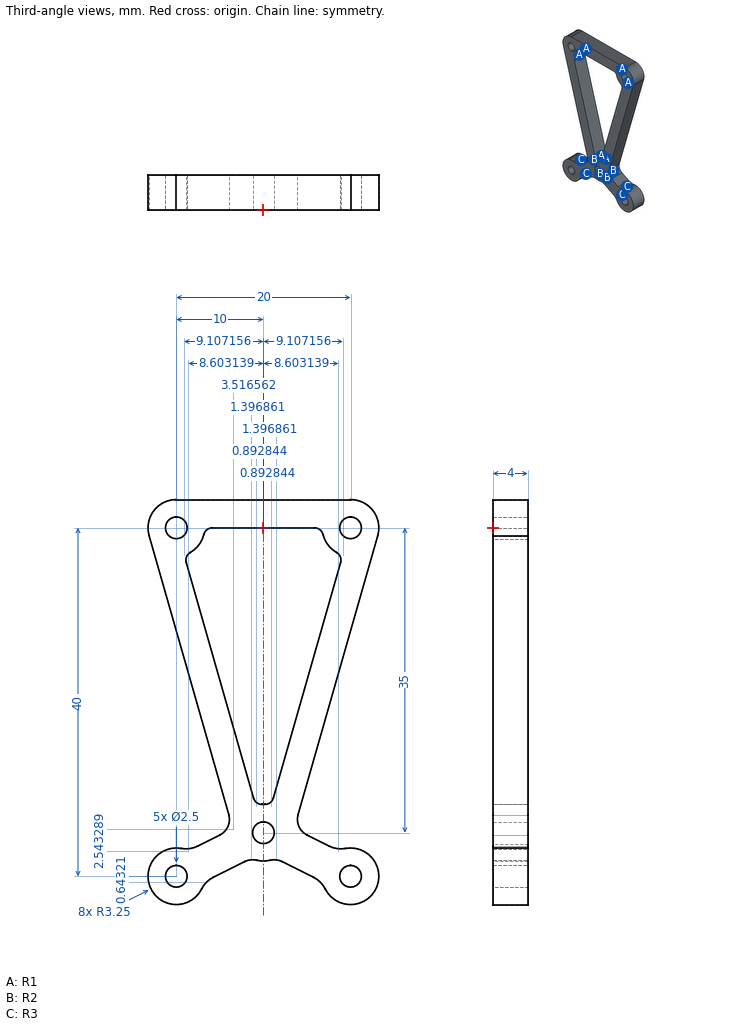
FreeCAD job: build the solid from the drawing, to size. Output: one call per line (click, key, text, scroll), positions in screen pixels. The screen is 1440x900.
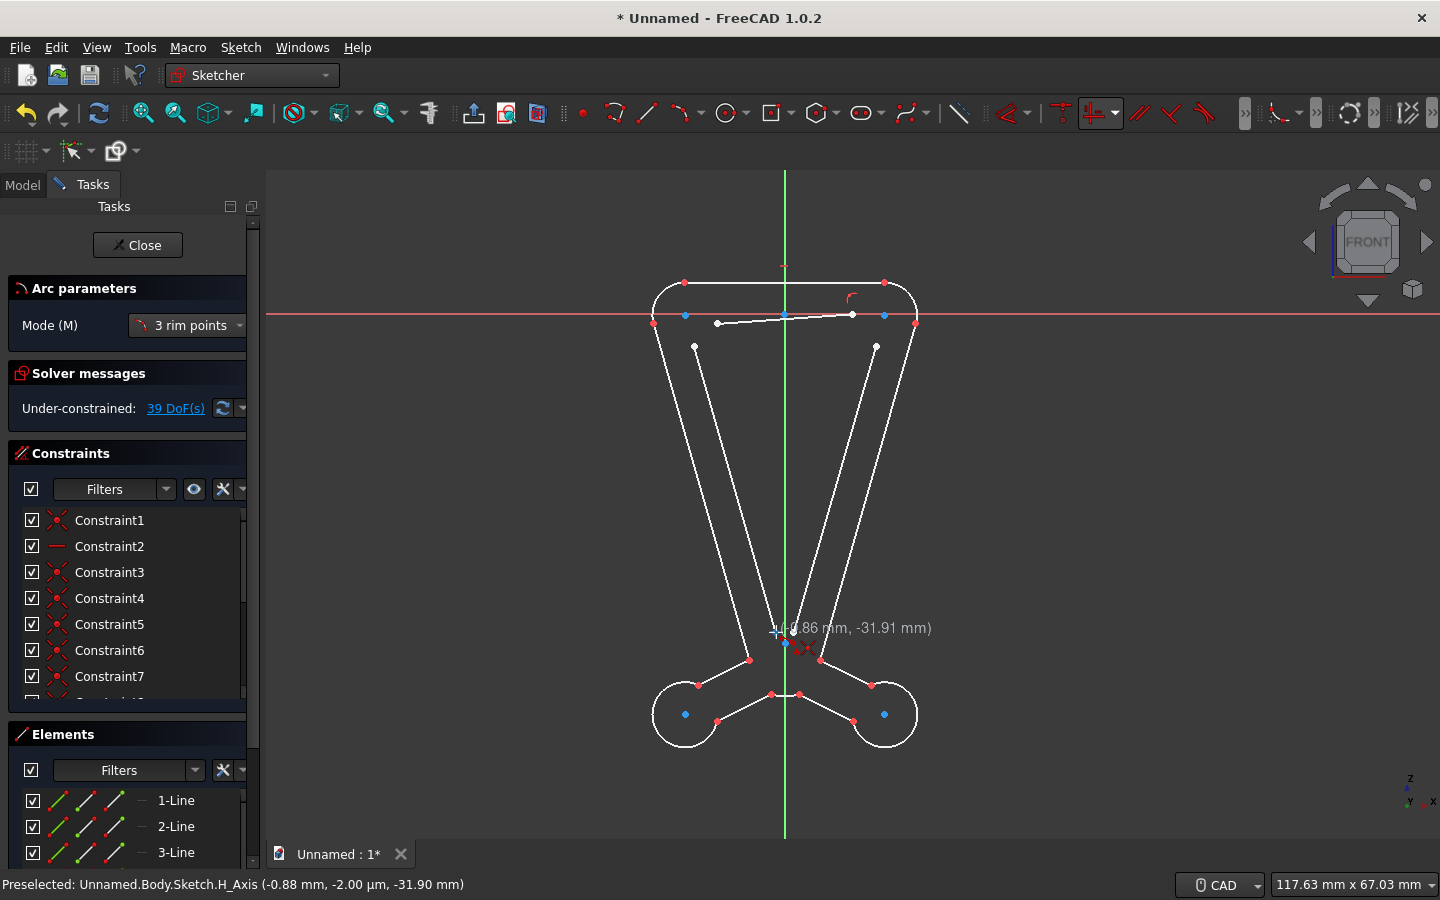
click(876, 347)
click(852, 314)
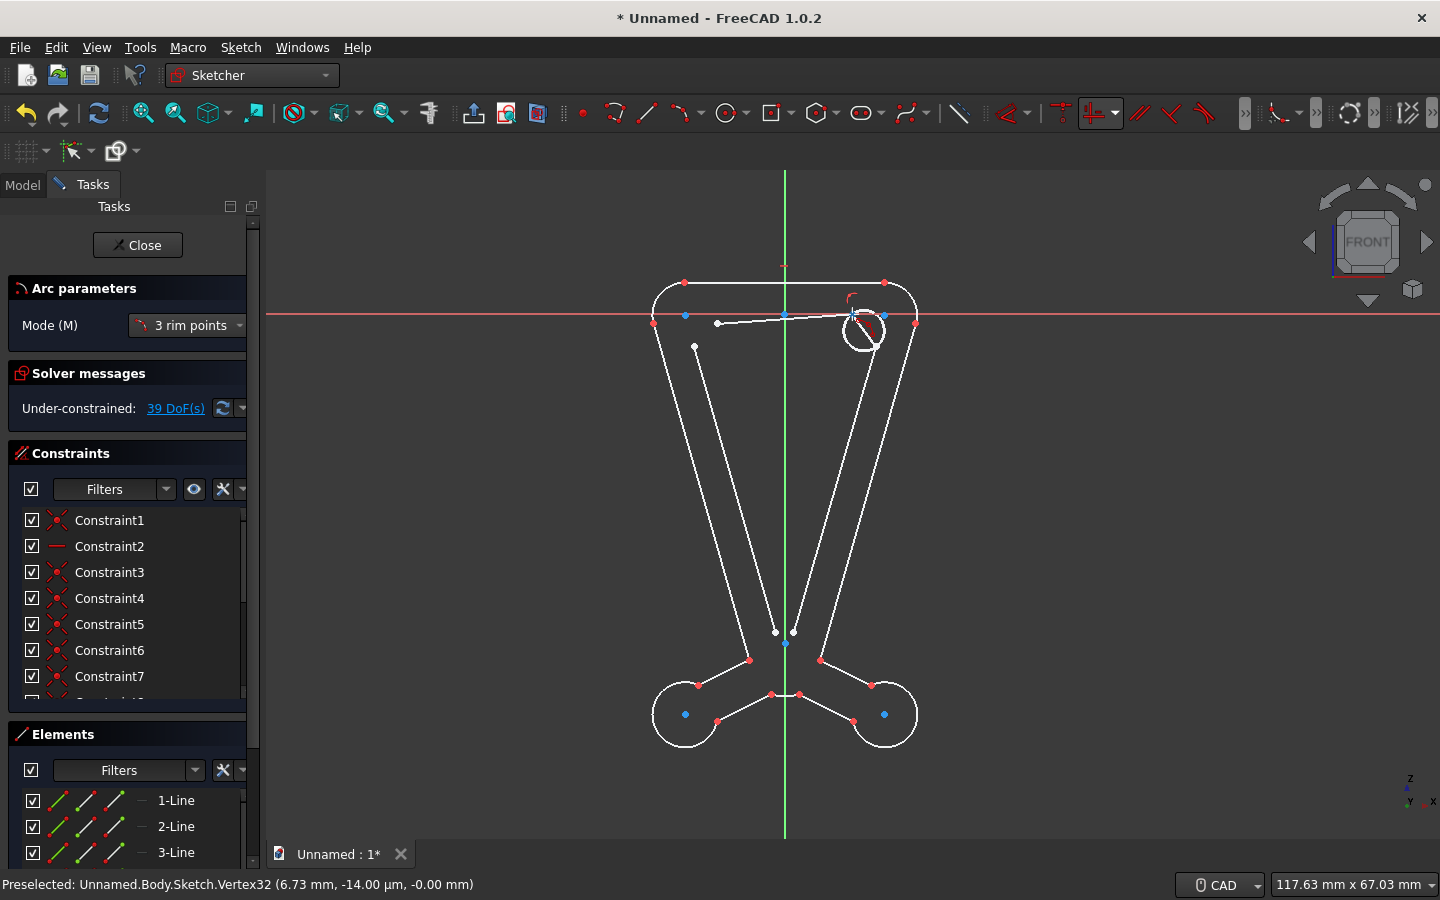
scroll(859, 334, up, 5)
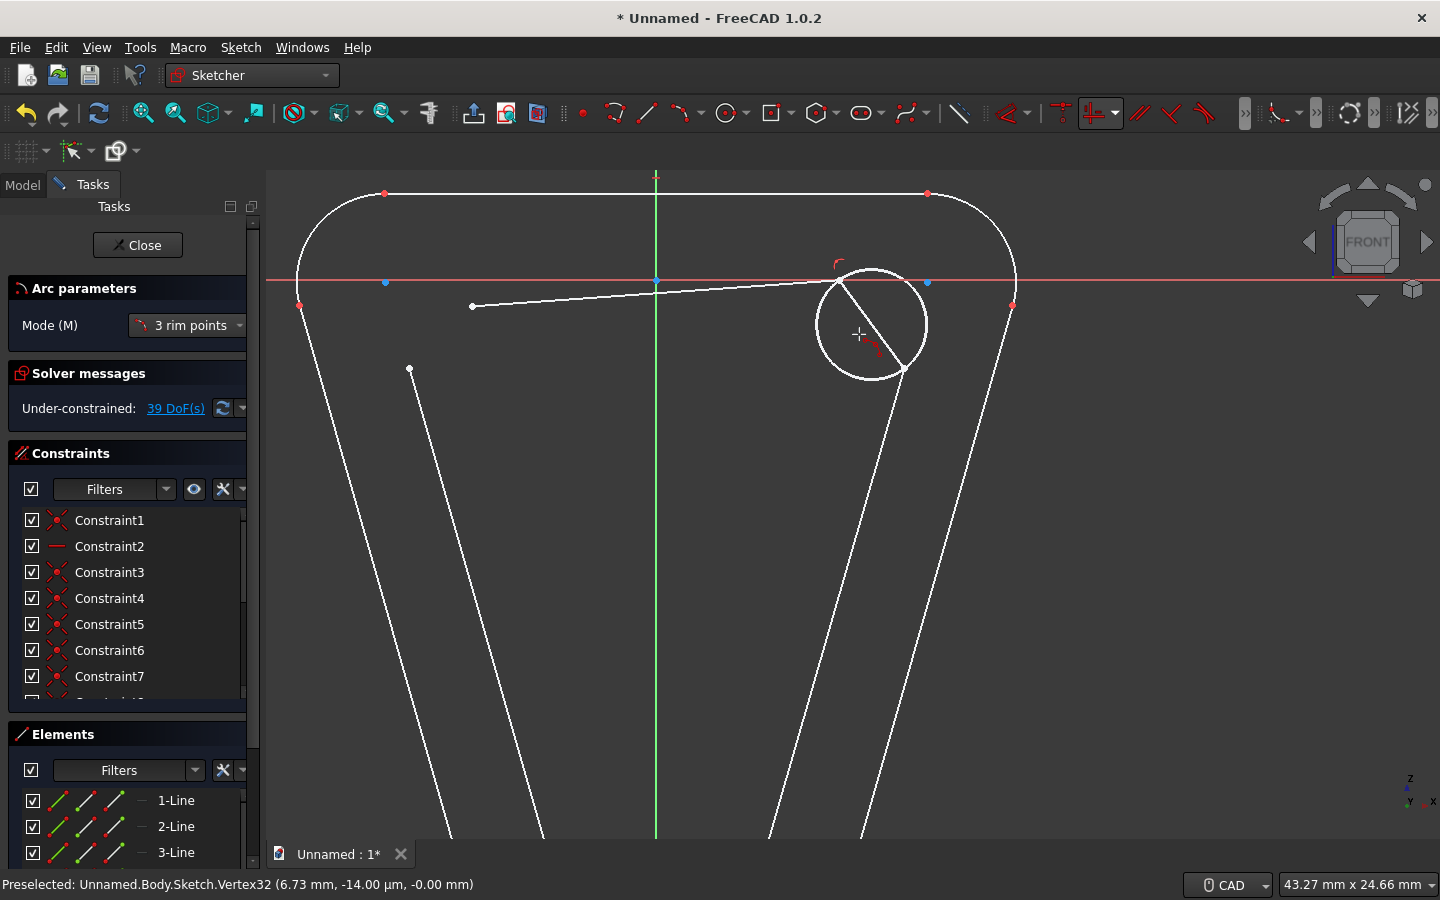
click(857, 333)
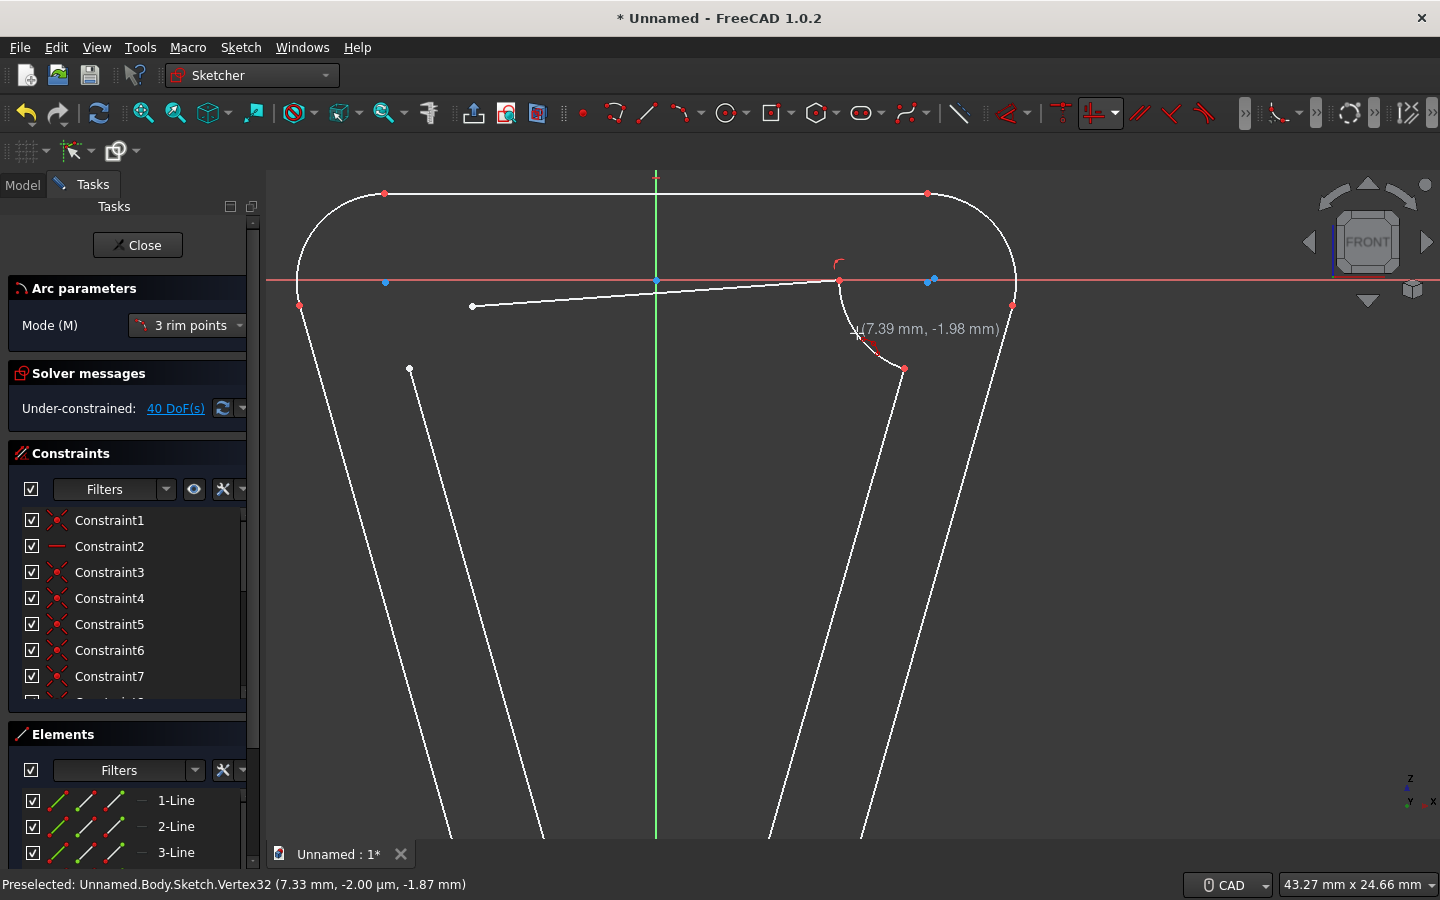
click(472, 306)
click(410, 369)
click(455, 333)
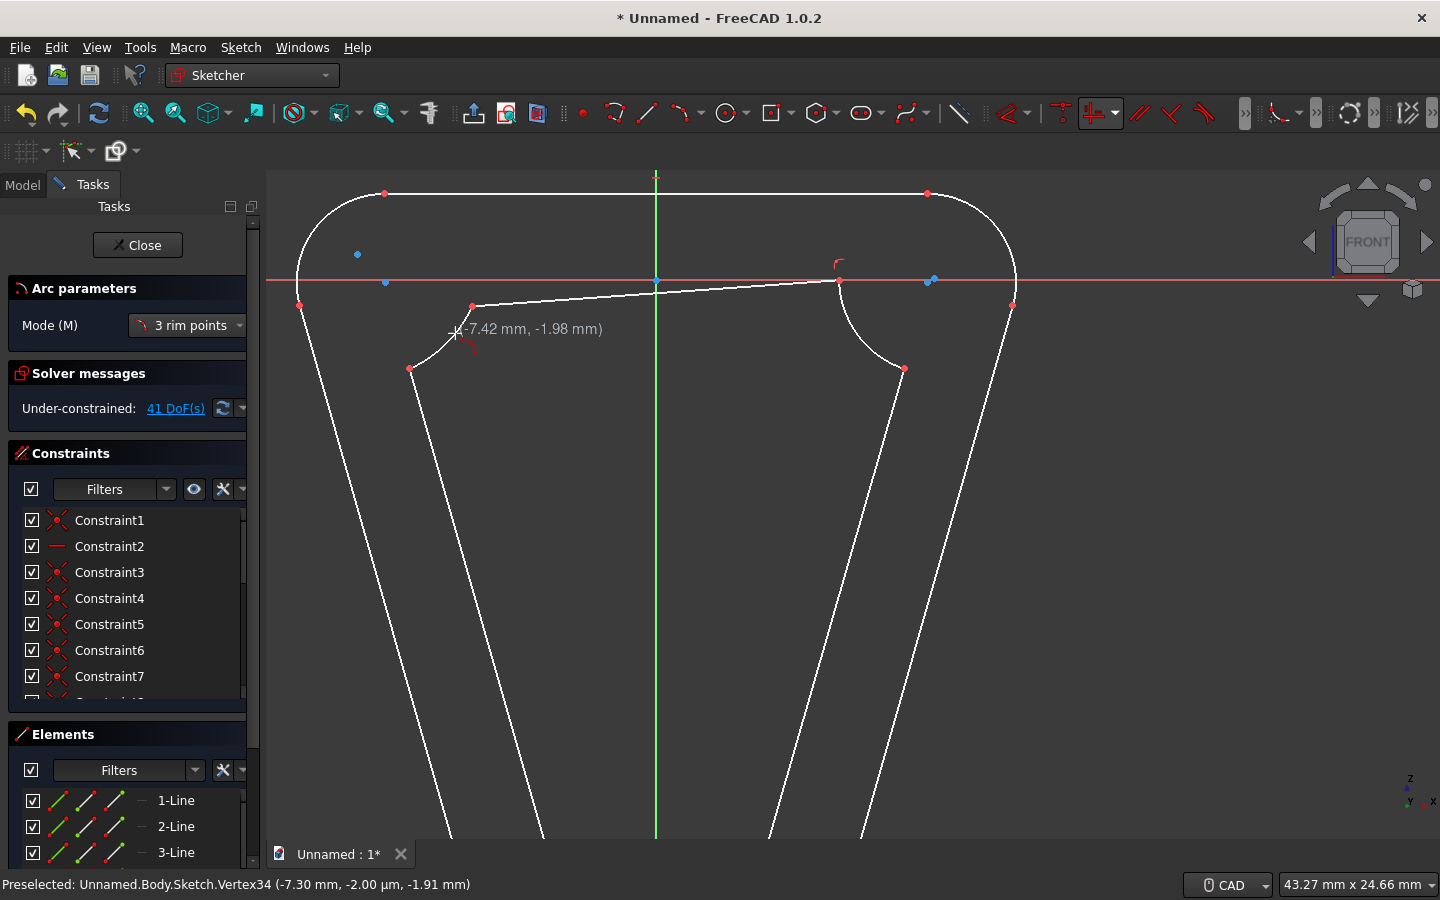
scroll(859, 333, down, 5)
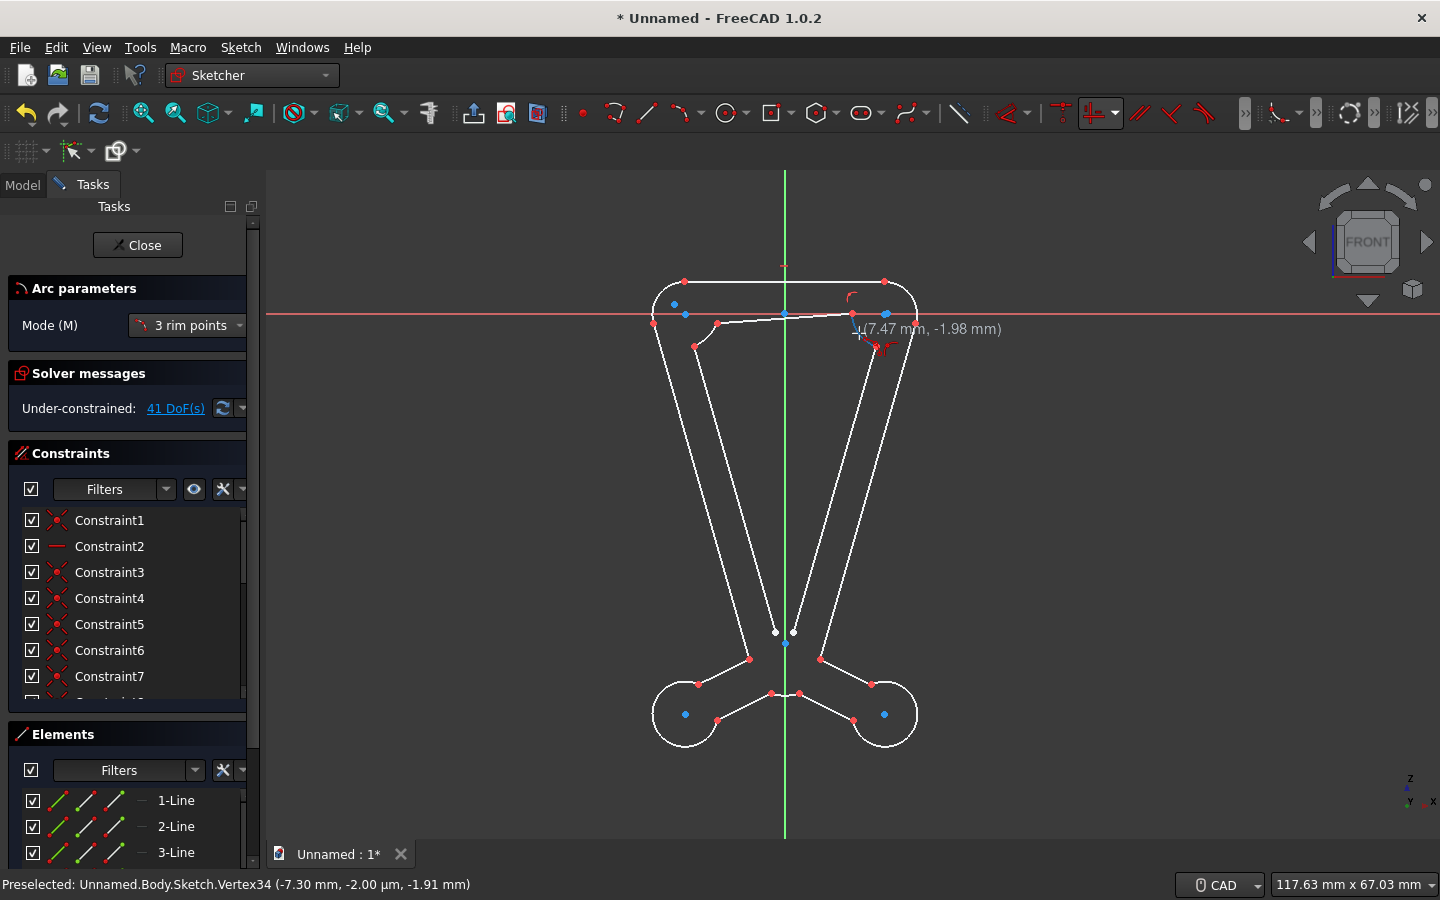
scroll(776, 632, up, 3)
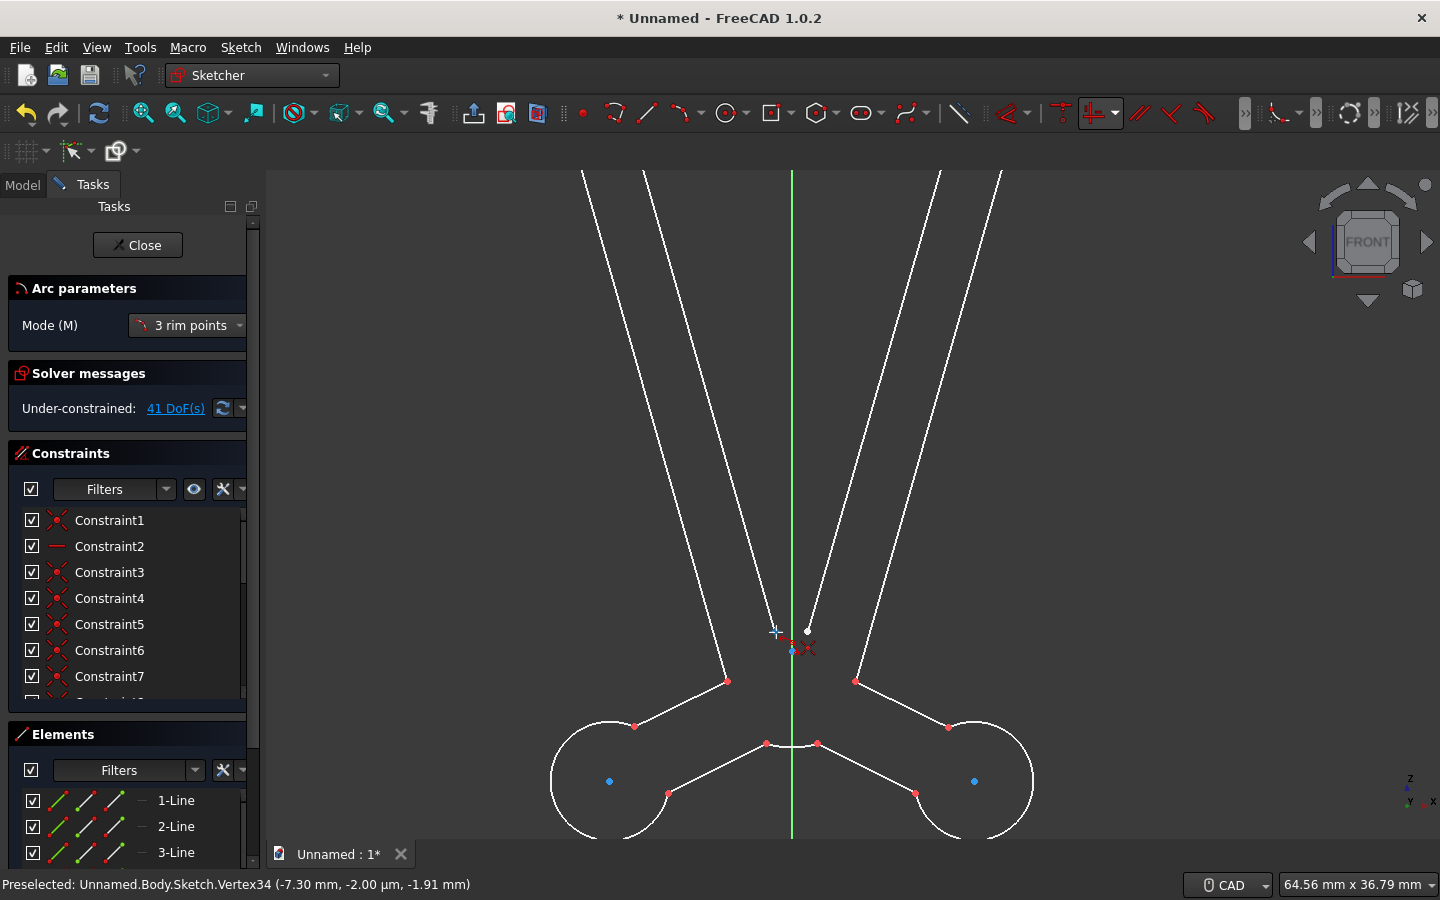
click(775, 632)
click(808, 632)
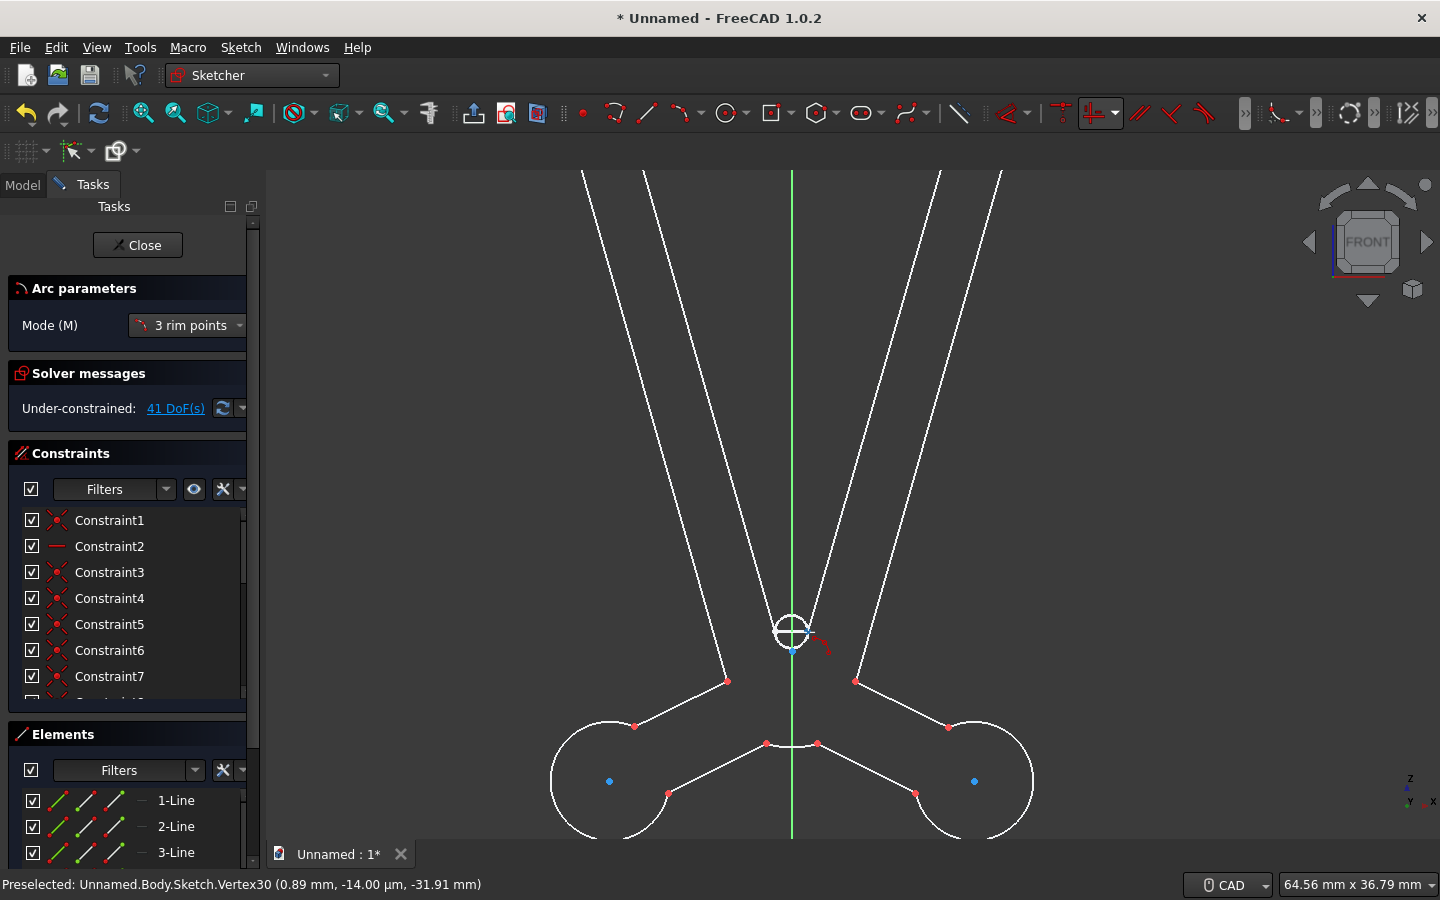
scroll(795, 629, up, 10)